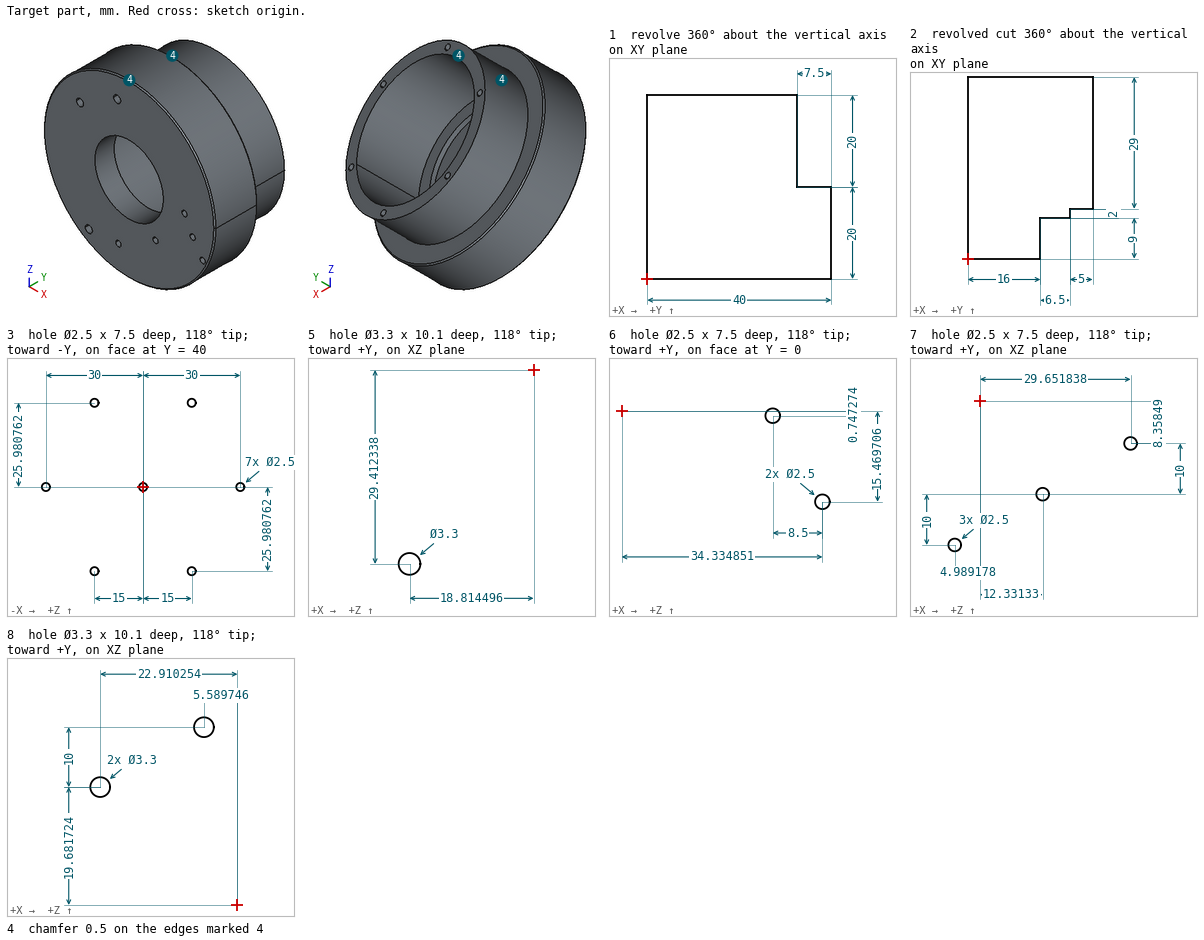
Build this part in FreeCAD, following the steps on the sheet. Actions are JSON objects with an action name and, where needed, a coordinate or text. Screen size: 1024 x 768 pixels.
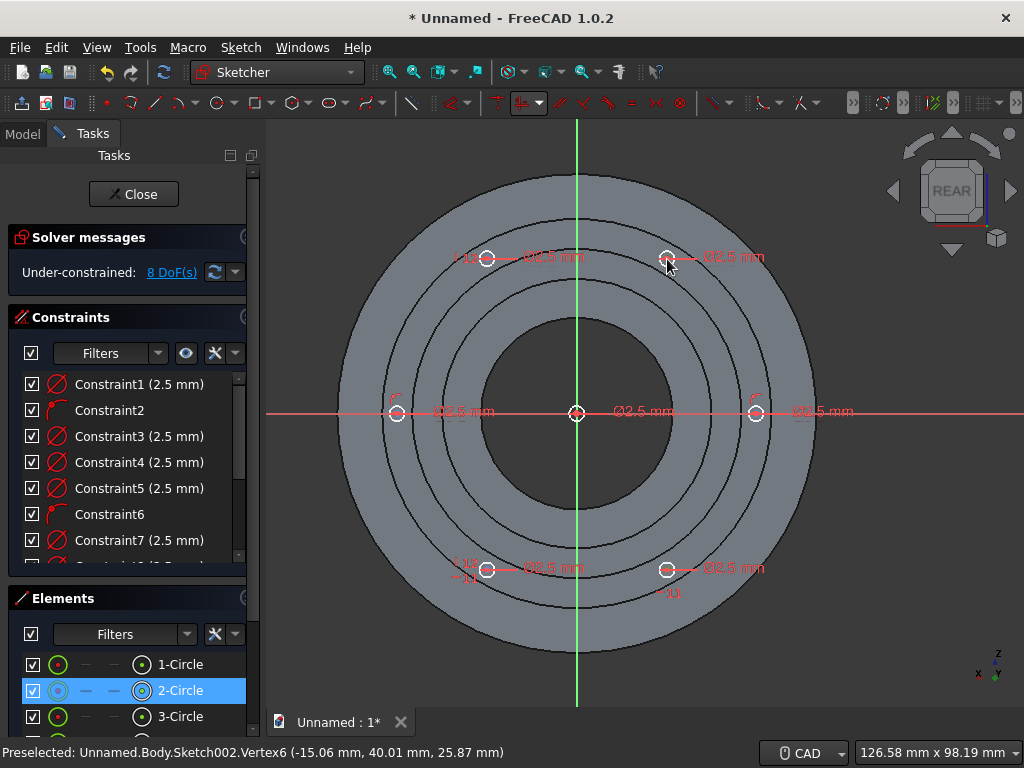
{"action": "key", "text": "v"}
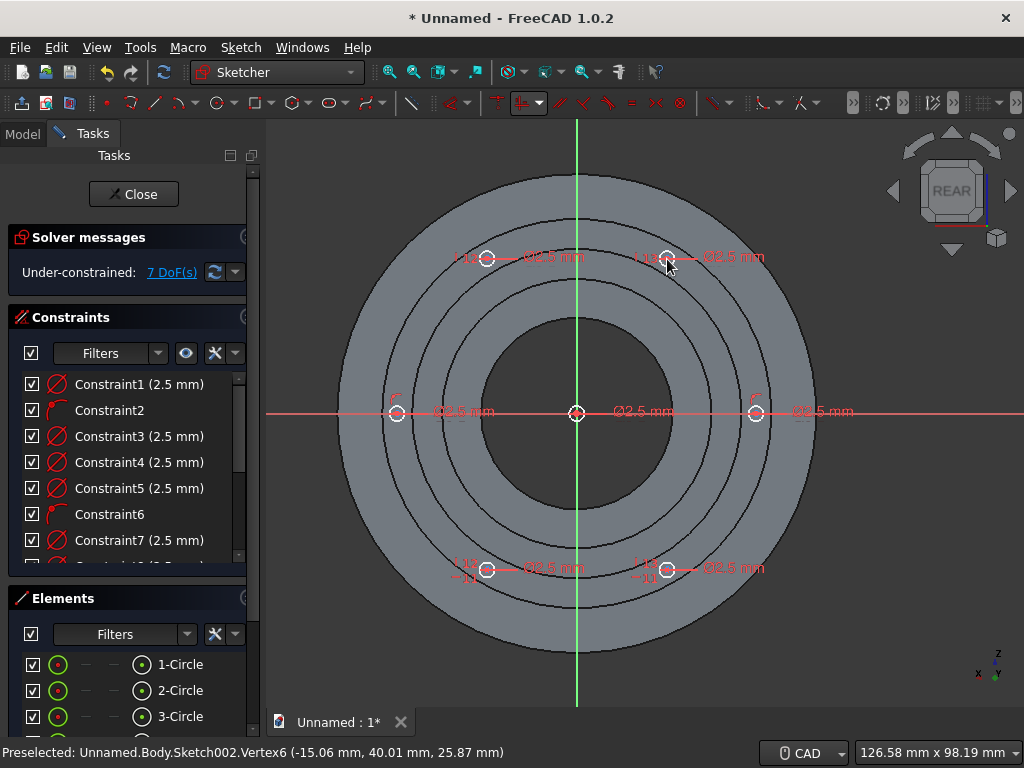
{"action": "left_click", "coordinate": [487, 259]}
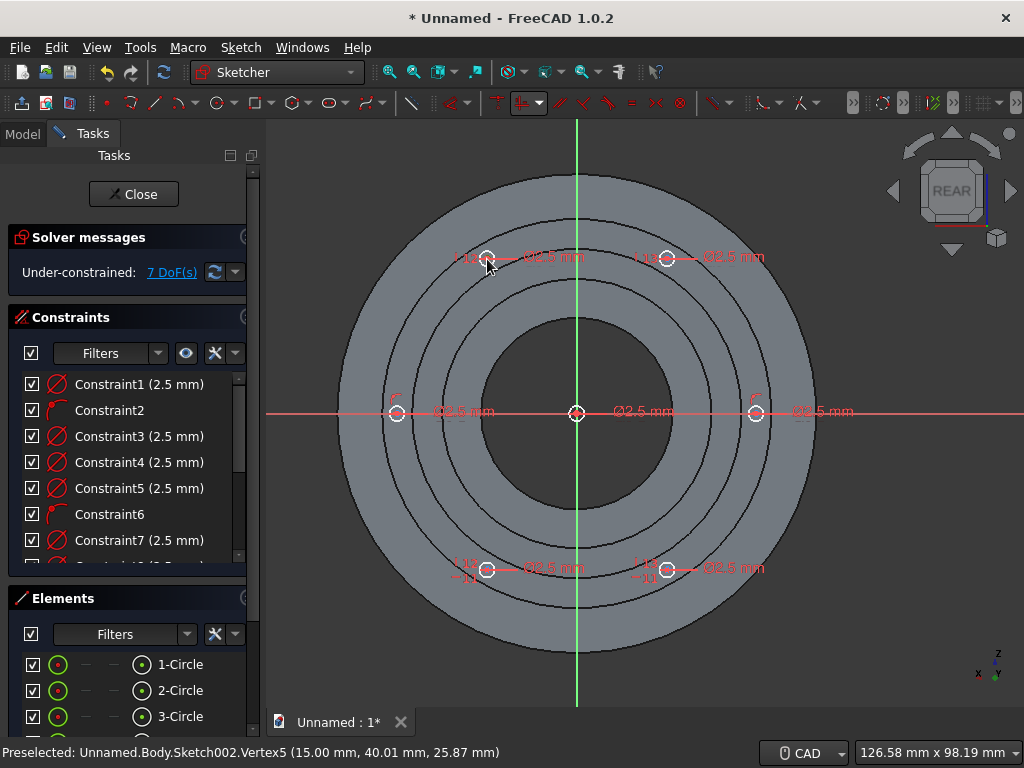
{"action": "left_click", "coordinate": [667, 259]}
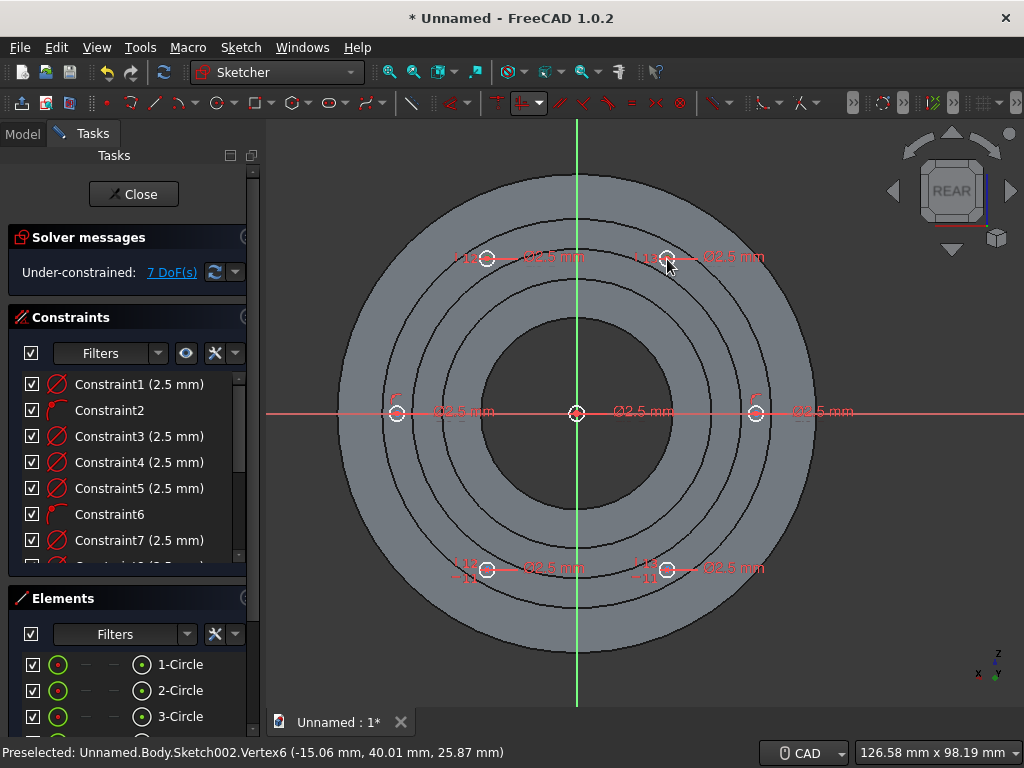
{"action": "left_click", "coordinate": [542, 104]}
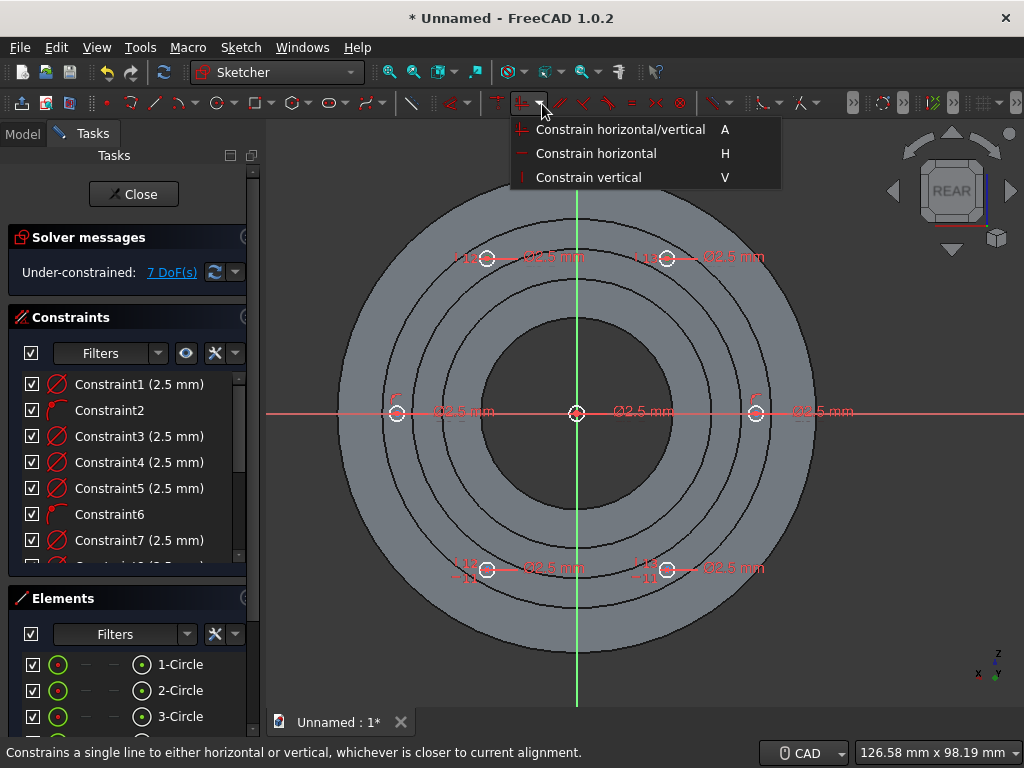
{"action": "left_click", "coordinate": [646, 153]}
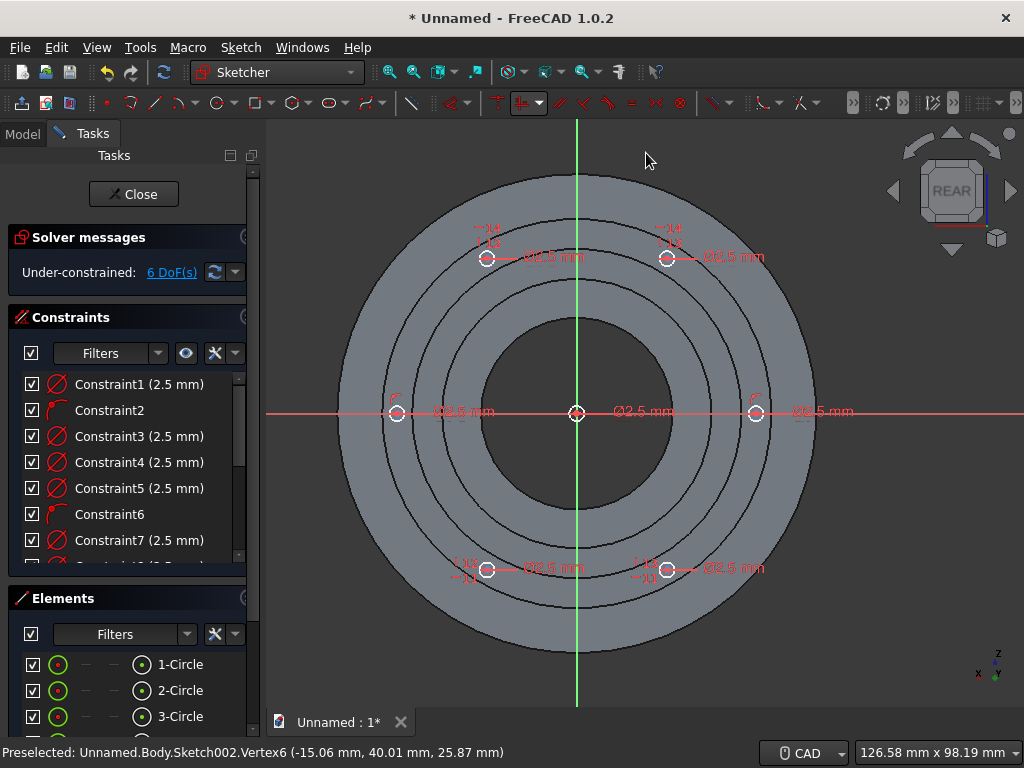
{"action": "left_click", "coordinate": [450, 104]}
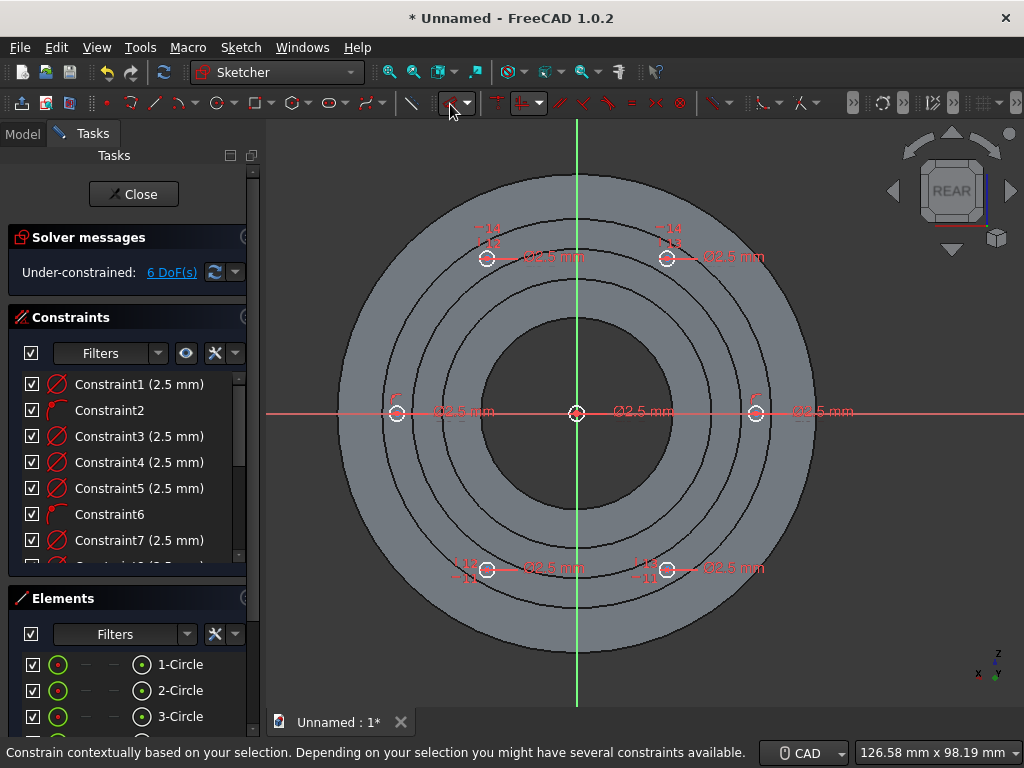
{"action": "left_click", "coordinate": [756, 414]}
{"action": "left_click", "coordinate": [666, 448]}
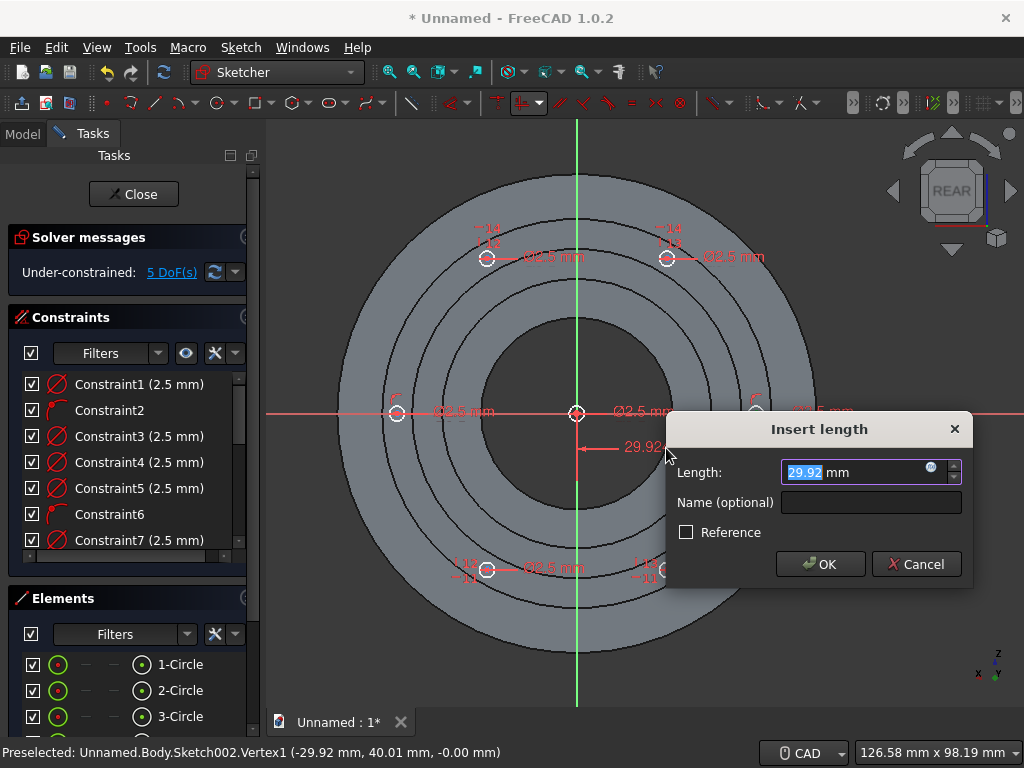
{"action": "type", "text": "30"}
{"action": "key", "text": "Return"}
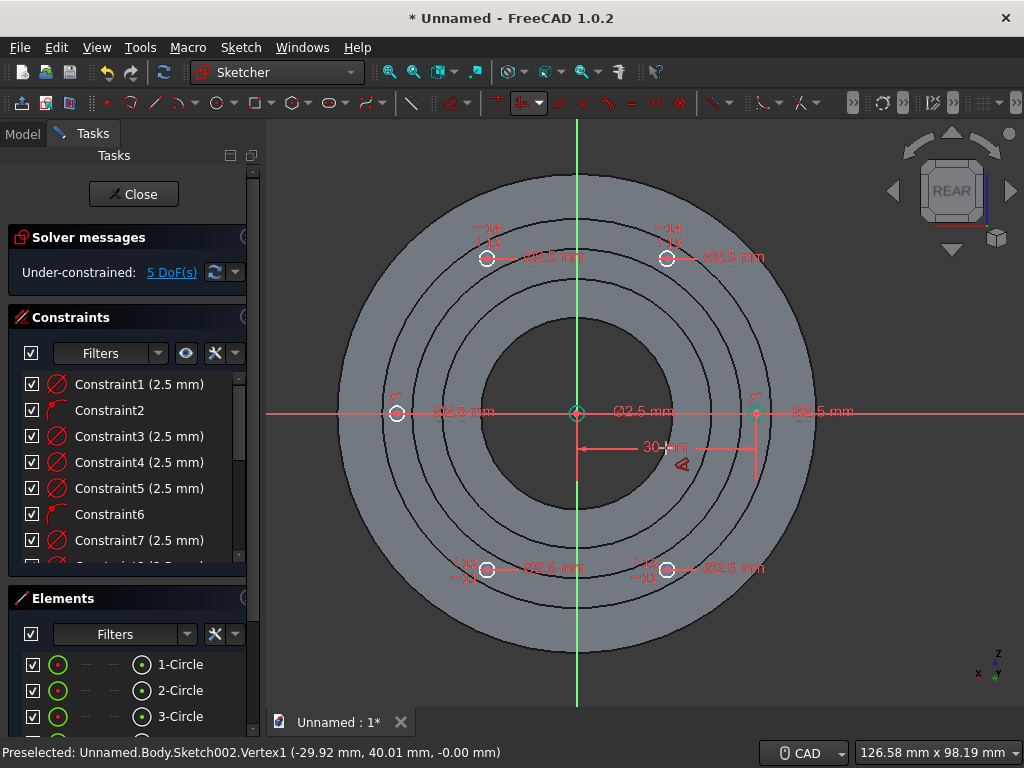
{"action": "left_click", "coordinate": [667, 570]}
{"action": "left_click", "coordinate": [622, 604]}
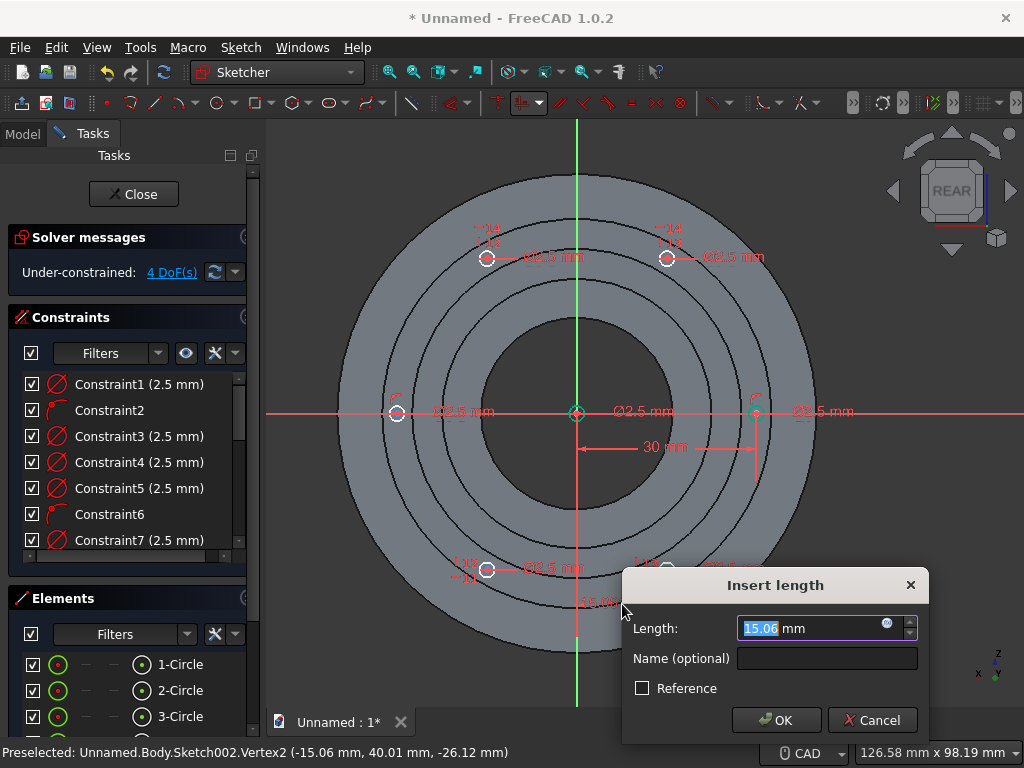
{"action": "type", "text": "15"}
{"action": "key", "text": "Return"}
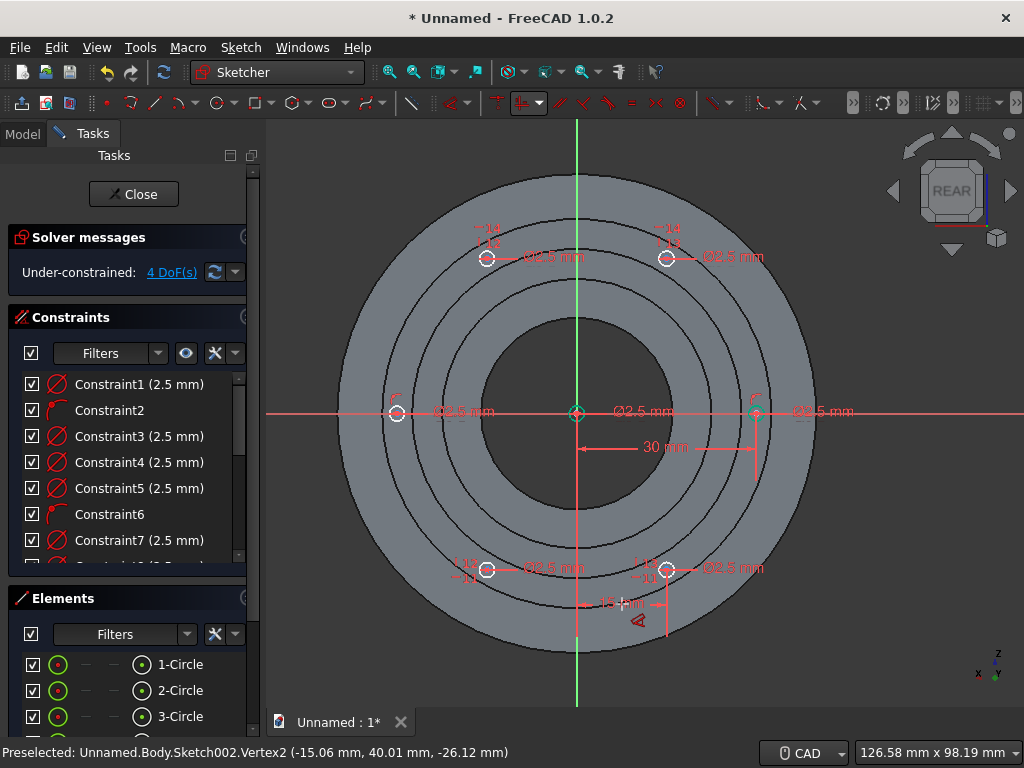
{"action": "left_click", "coordinate": [487, 570]}
{"action": "left_click", "coordinate": [532, 604]}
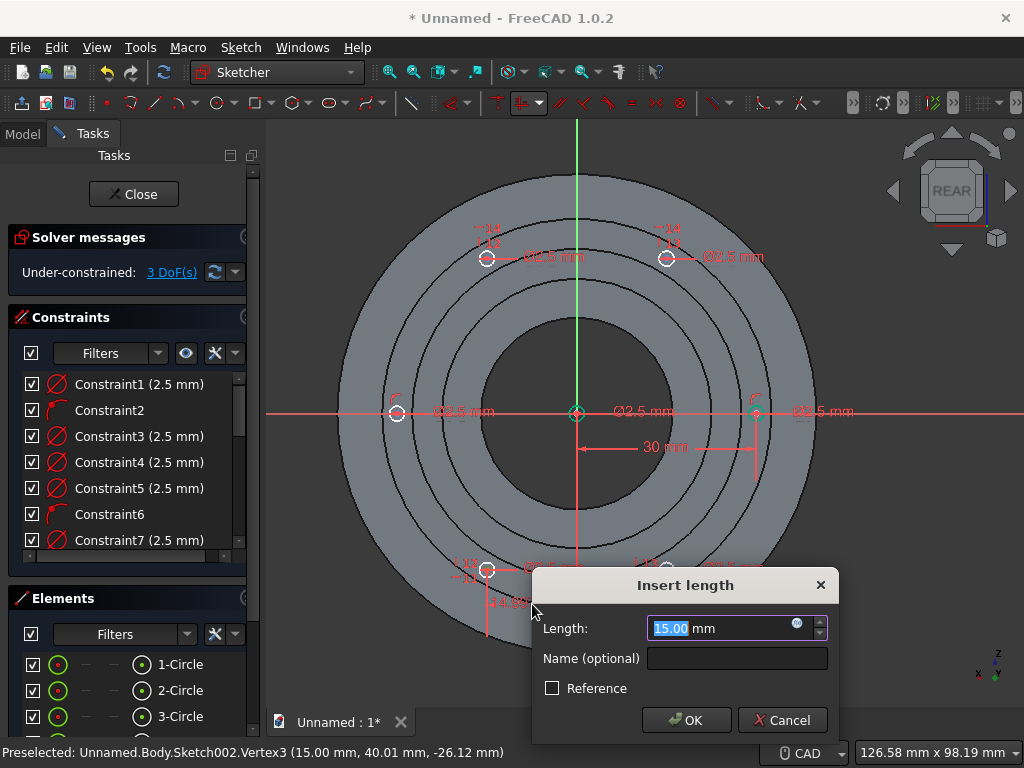
{"action": "type", "text": "15"}
{"action": "key", "text": "Return"}